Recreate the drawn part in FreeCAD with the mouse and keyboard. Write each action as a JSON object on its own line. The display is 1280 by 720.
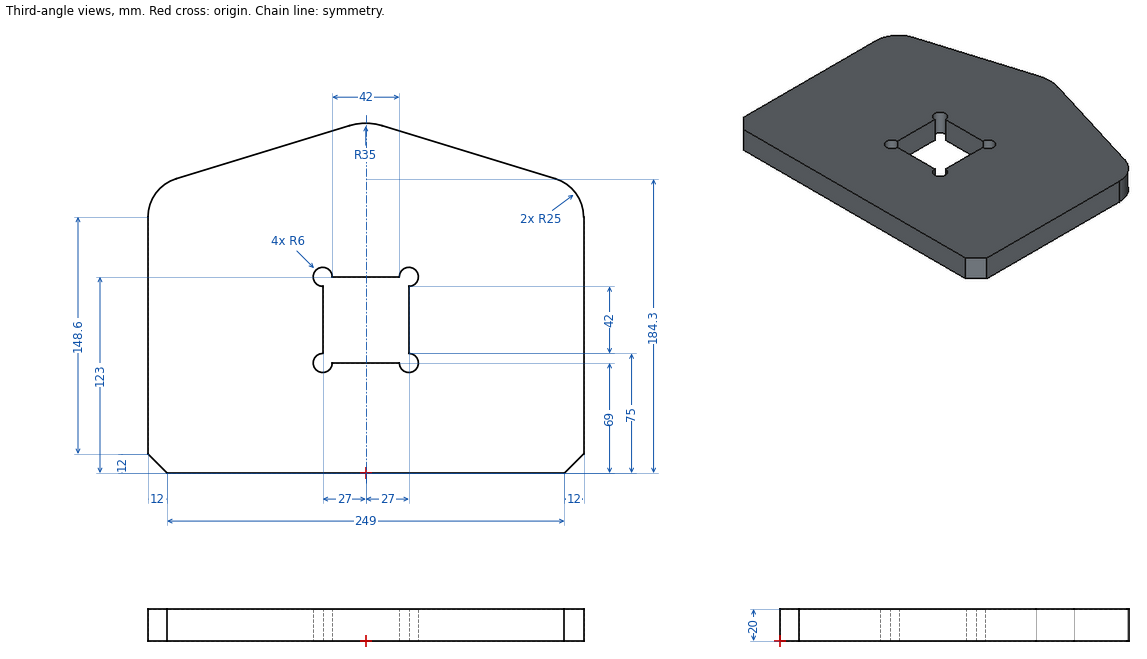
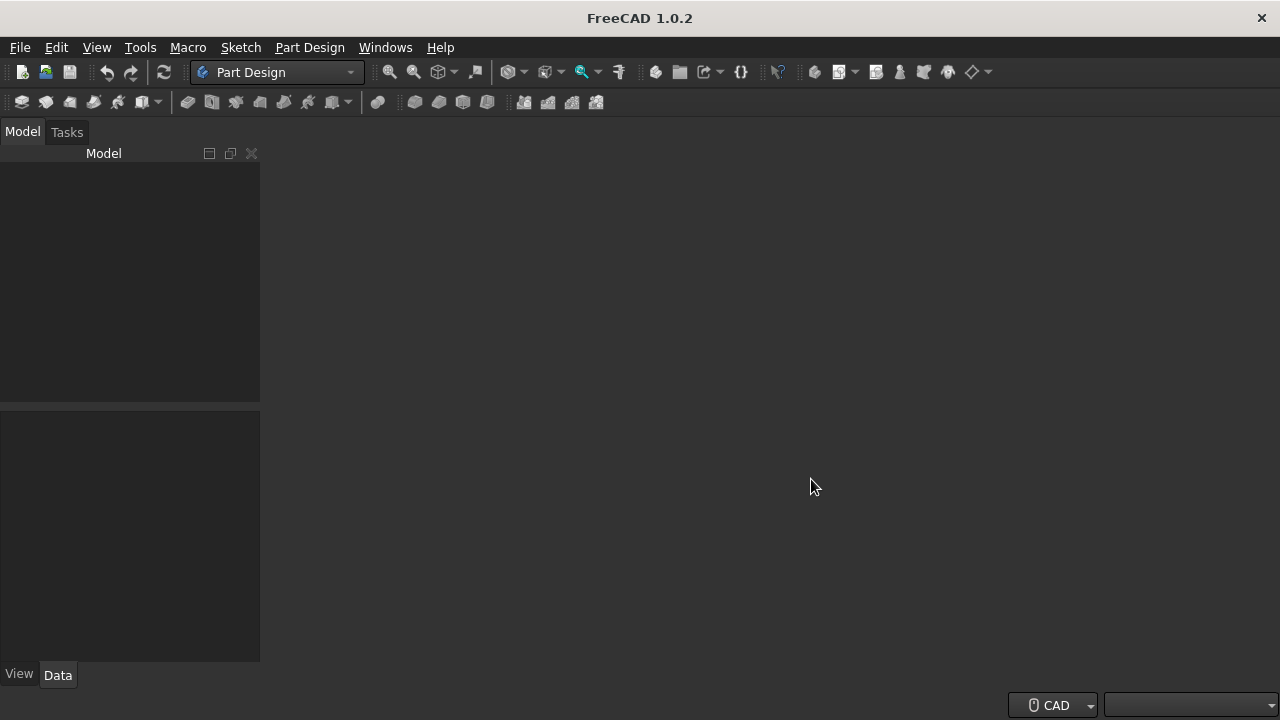
{"action": "left_click", "coordinate": [22, 72]}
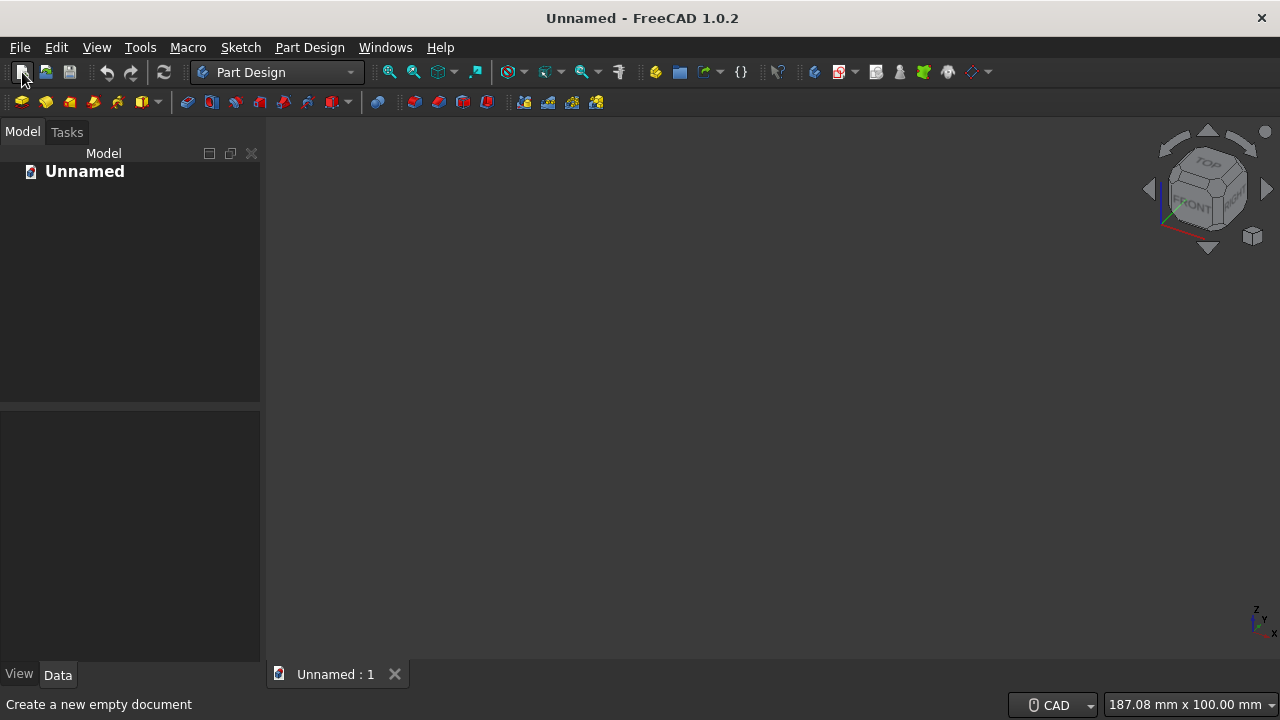
{"action": "left_click", "coordinate": [840, 72]}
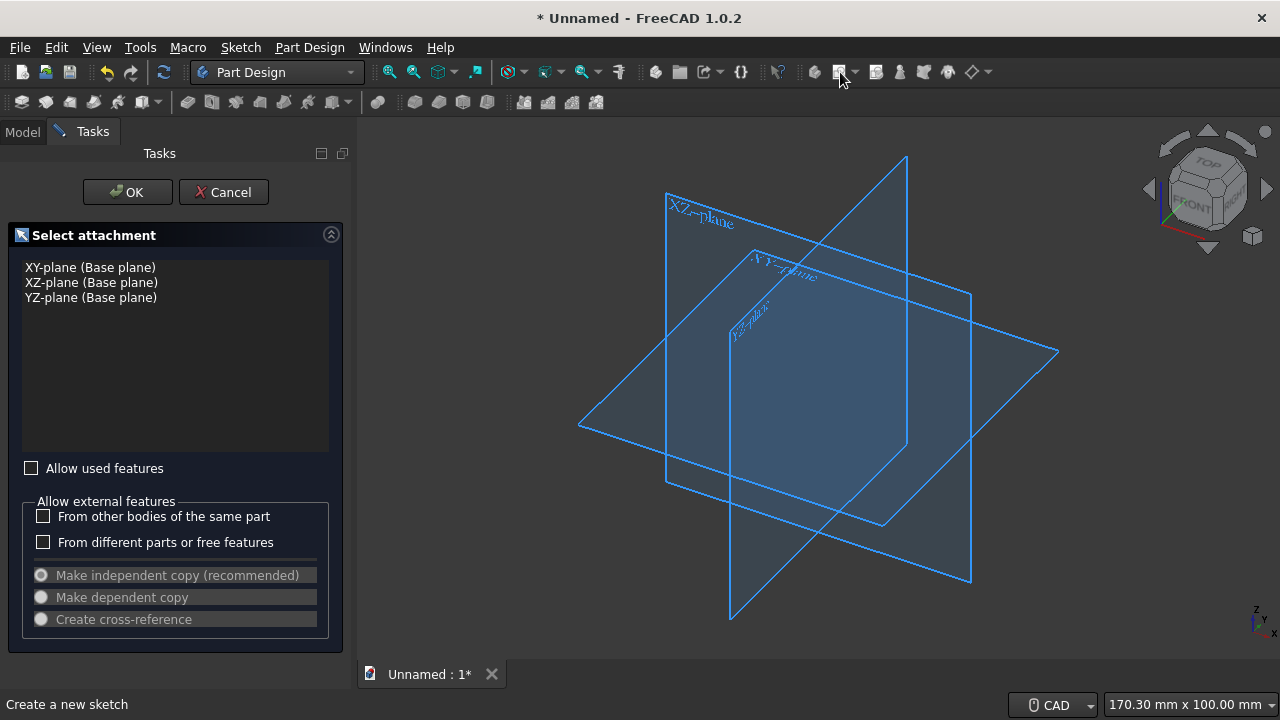
{"action": "left_click", "coordinate": [82, 268]}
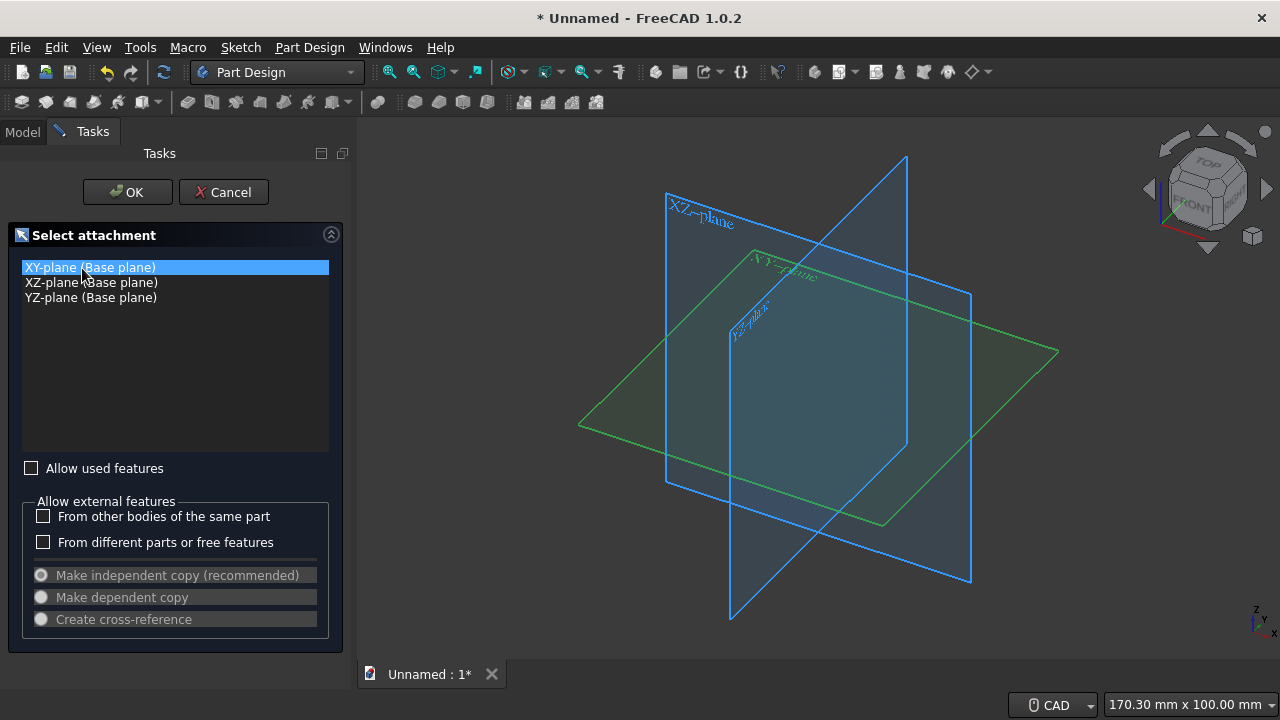
{"action": "left_click", "coordinate": [128, 192]}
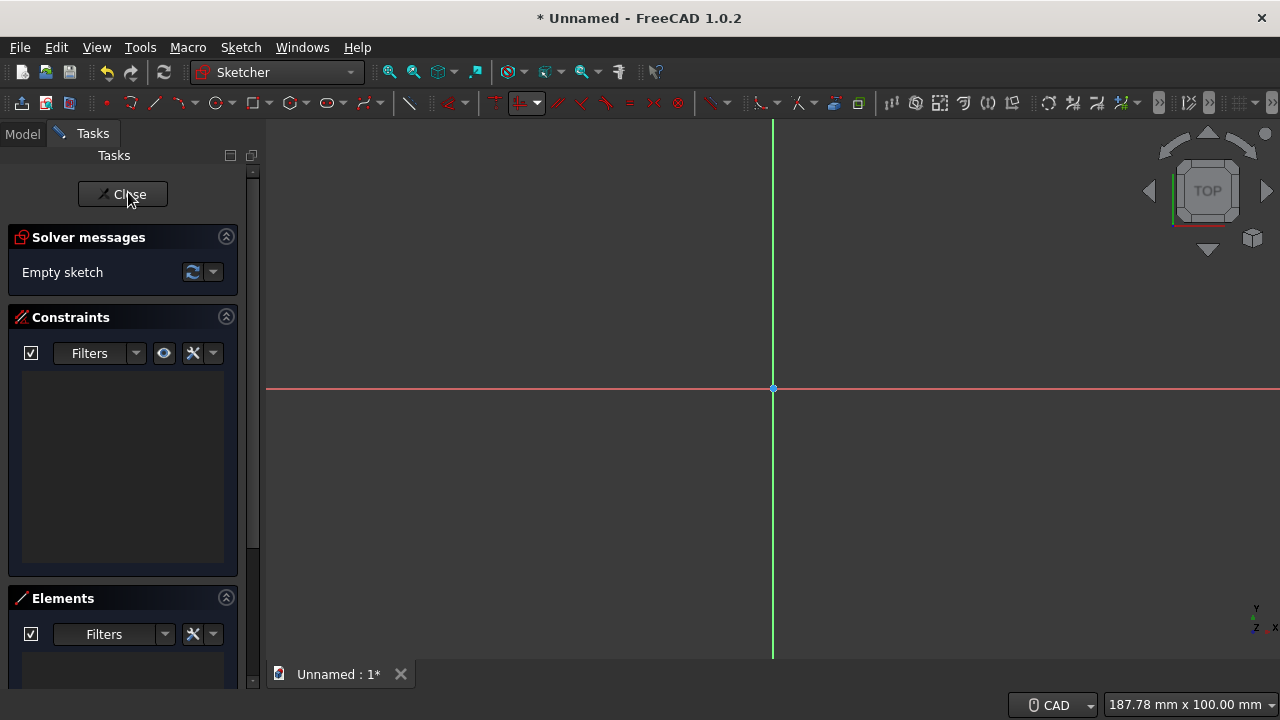
{"action": "scroll", "coordinate": [675, 631], "scroll_direction": "down", "scroll_amount": 6}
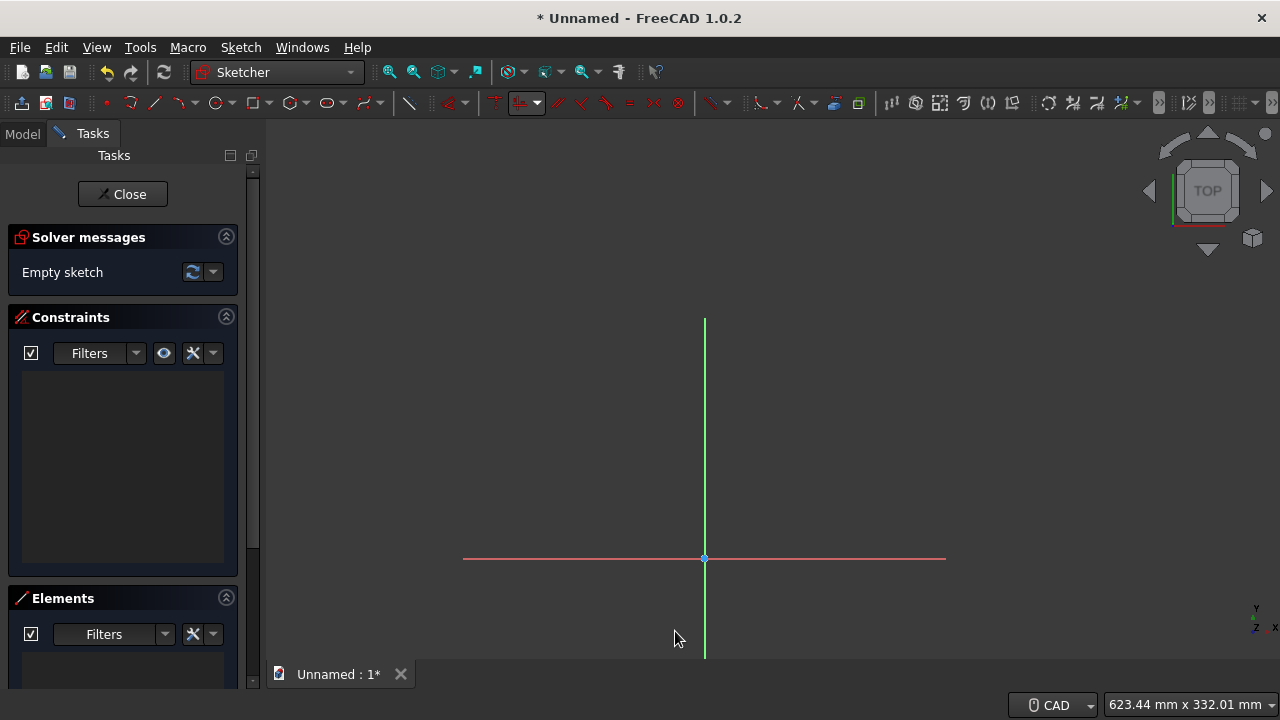
{"action": "left_click", "coordinate": [156, 104]}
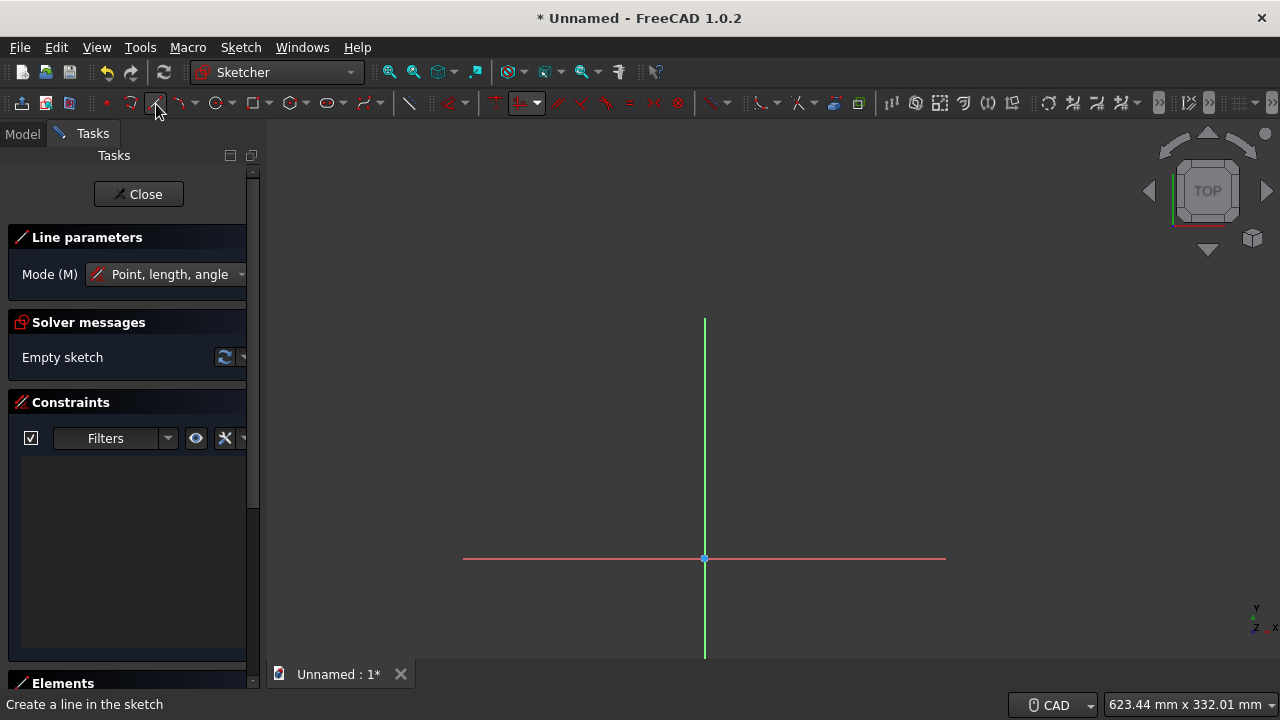
{"action": "left_click", "coordinate": [898, 259]}
{"action": "left_click", "coordinate": [721, 205]}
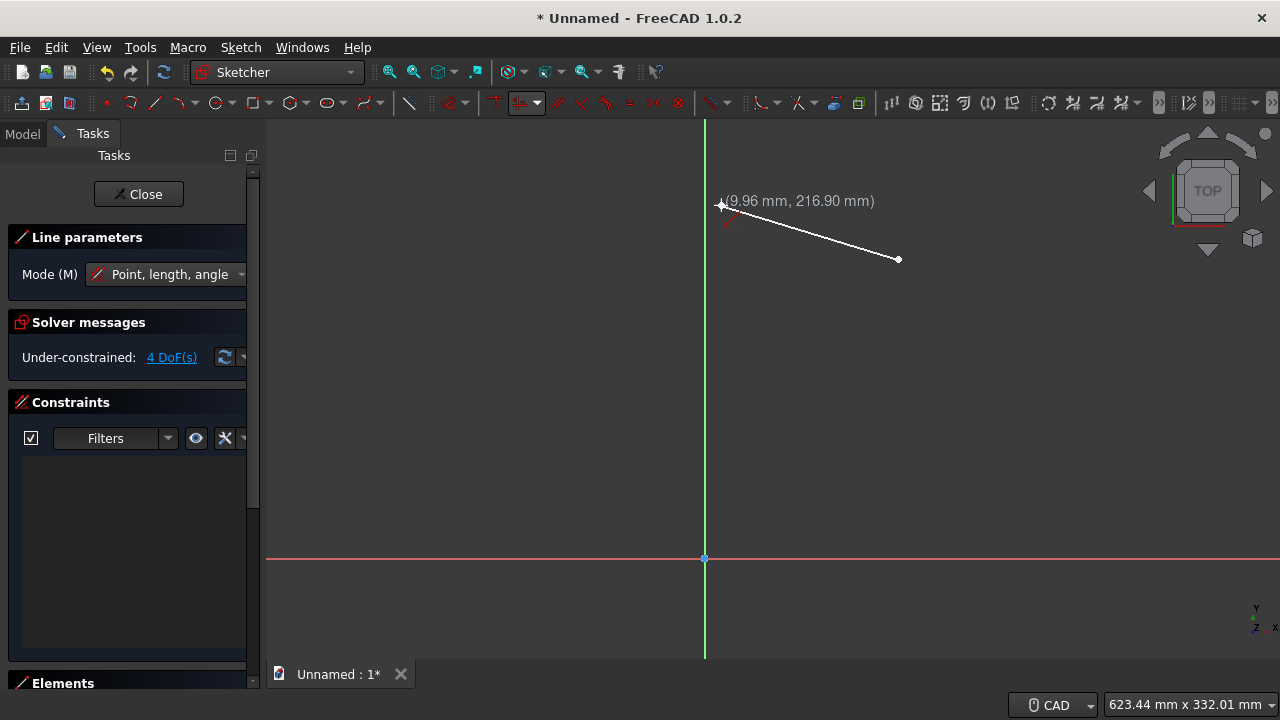
{"action": "left_click", "coordinate": [688, 205]}
{"action": "left_click", "coordinate": [512, 259]}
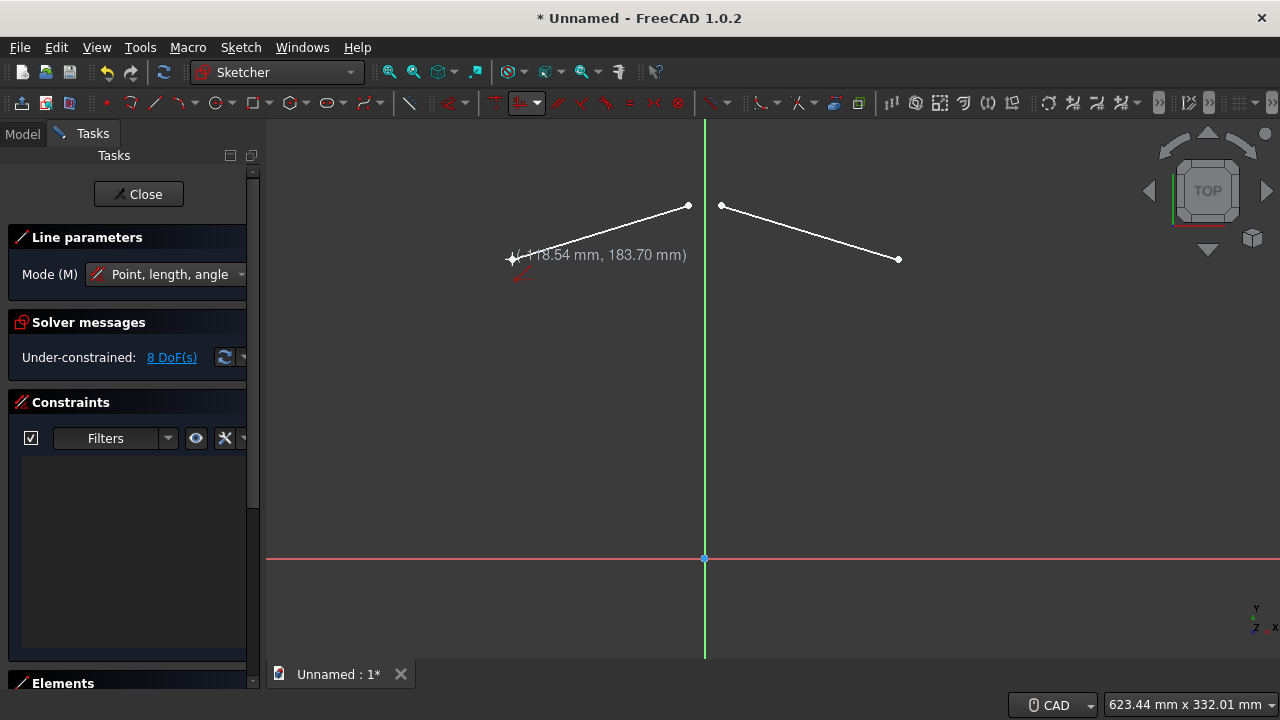
{"action": "left_click", "coordinate": [132, 104]}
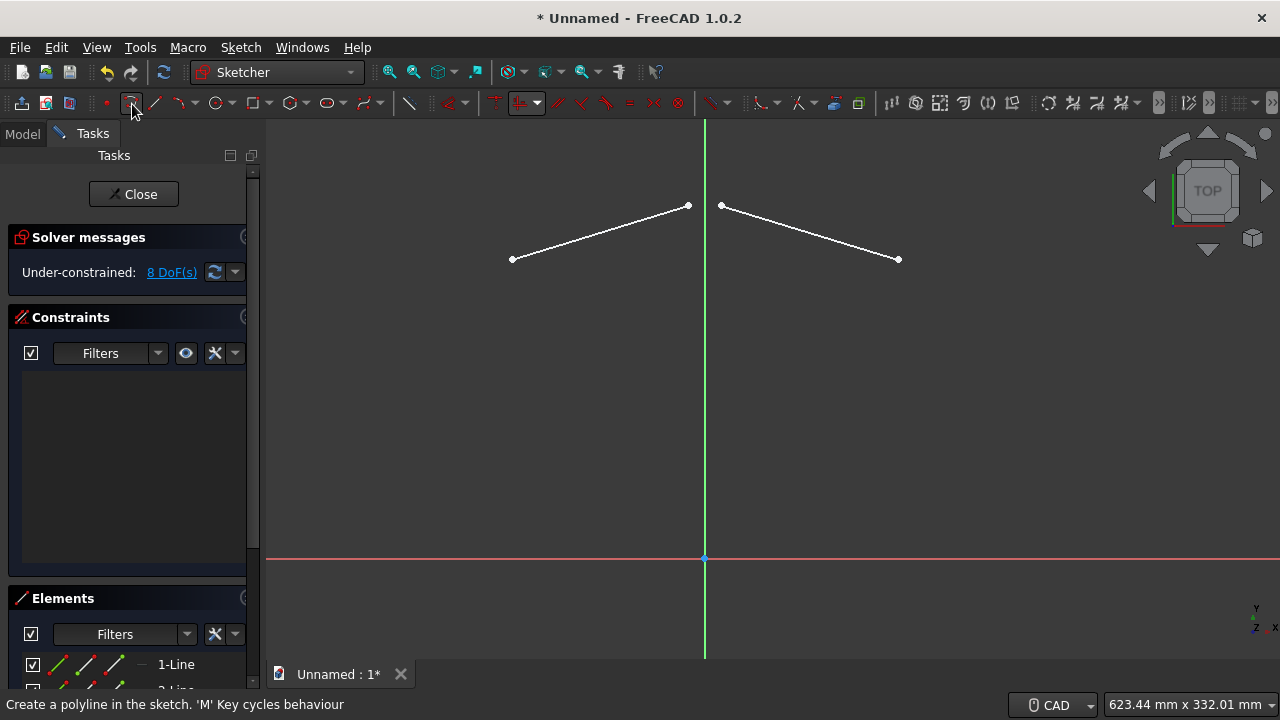
{"action": "left_click", "coordinate": [483, 298]}
{"action": "left_click", "coordinate": [483, 539]}
{"action": "left_click", "coordinate": [502, 559]}
{"action": "left_click", "coordinate": [907, 550]}
{"action": "left_click", "coordinate": [927, 539]}
{"action": "left_click", "coordinate": [927, 298]}
{"action": "right_click", "coordinate": [927, 298]}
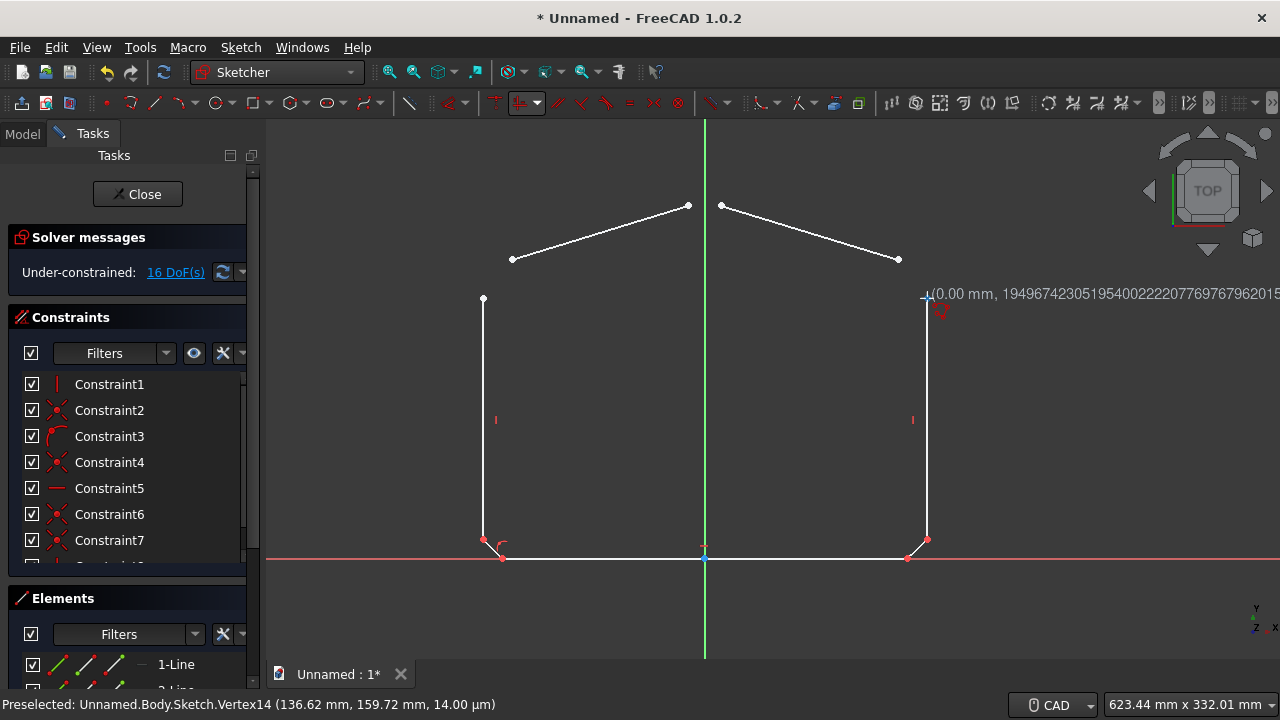
{"action": "left_click", "coordinate": [180, 104]}